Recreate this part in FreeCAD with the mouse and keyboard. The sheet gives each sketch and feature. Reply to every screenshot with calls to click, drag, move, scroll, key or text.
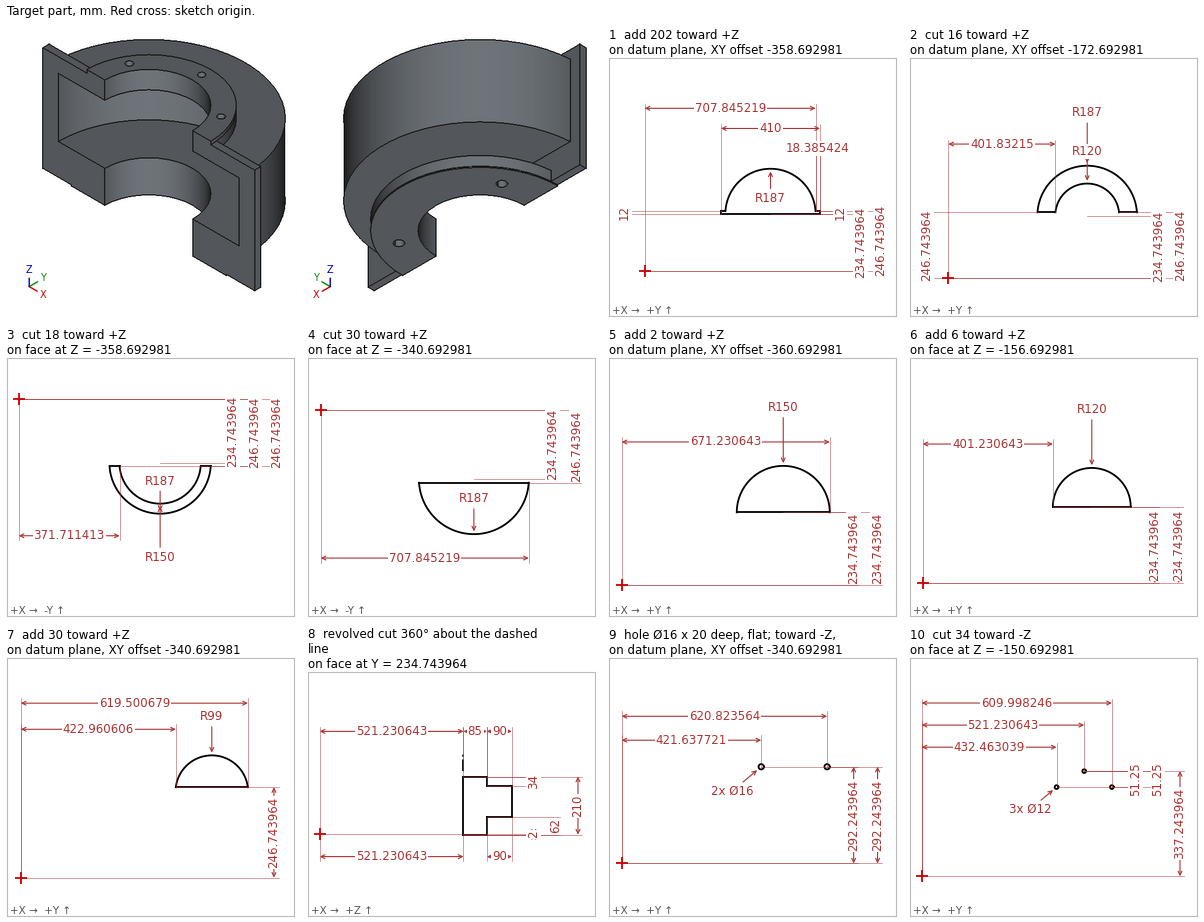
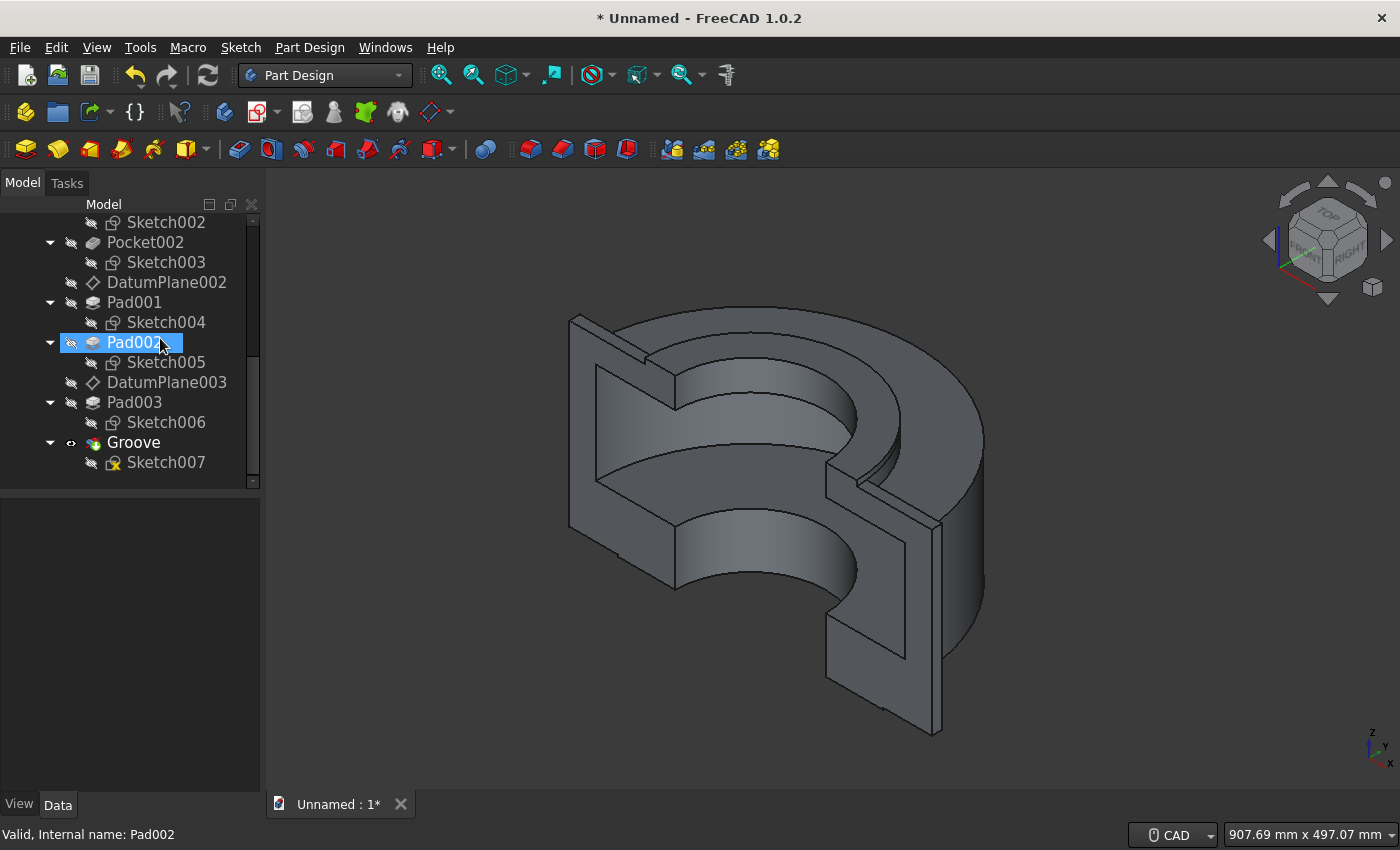
scroll(160, 338, up, 15)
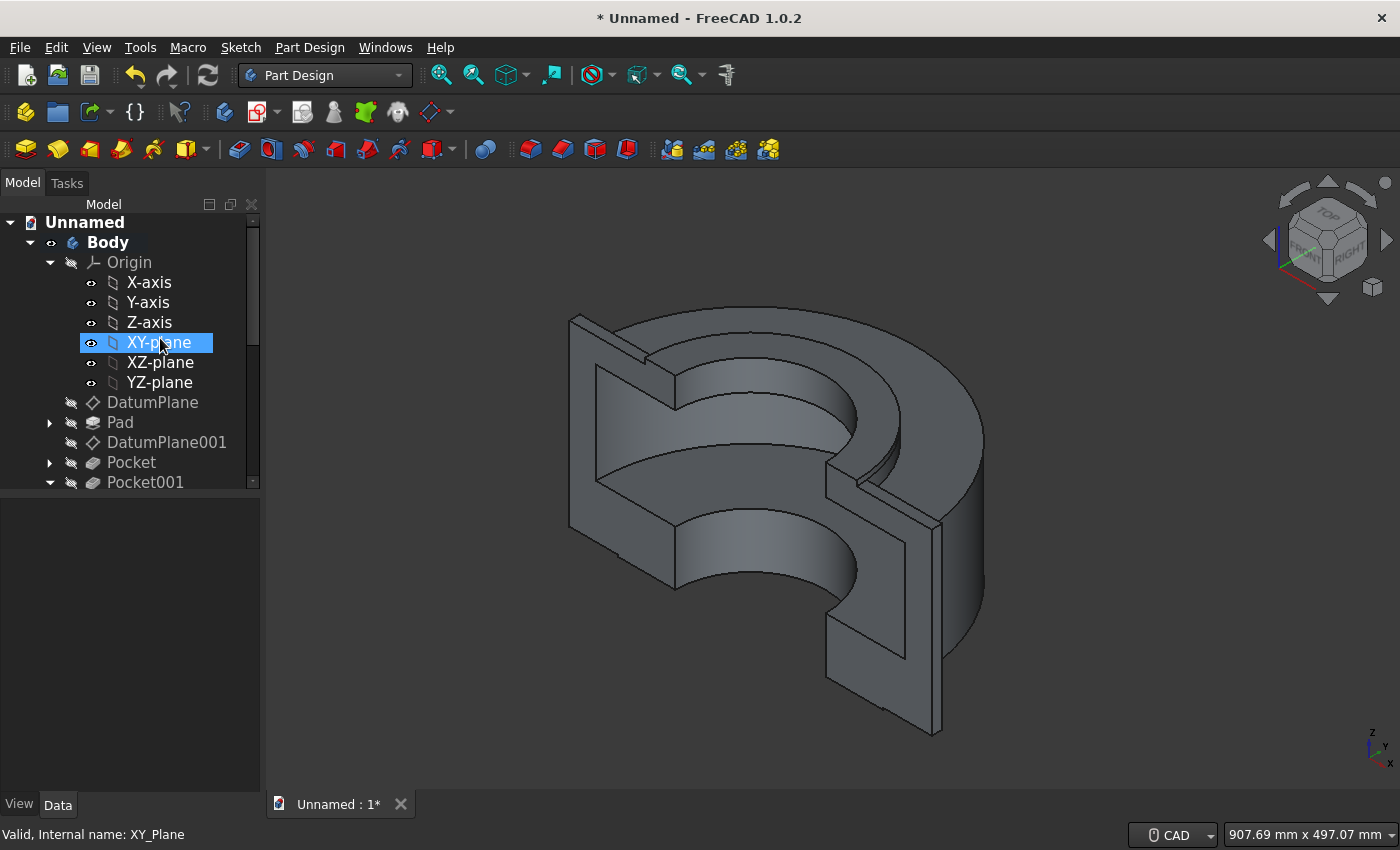
click(136, 343)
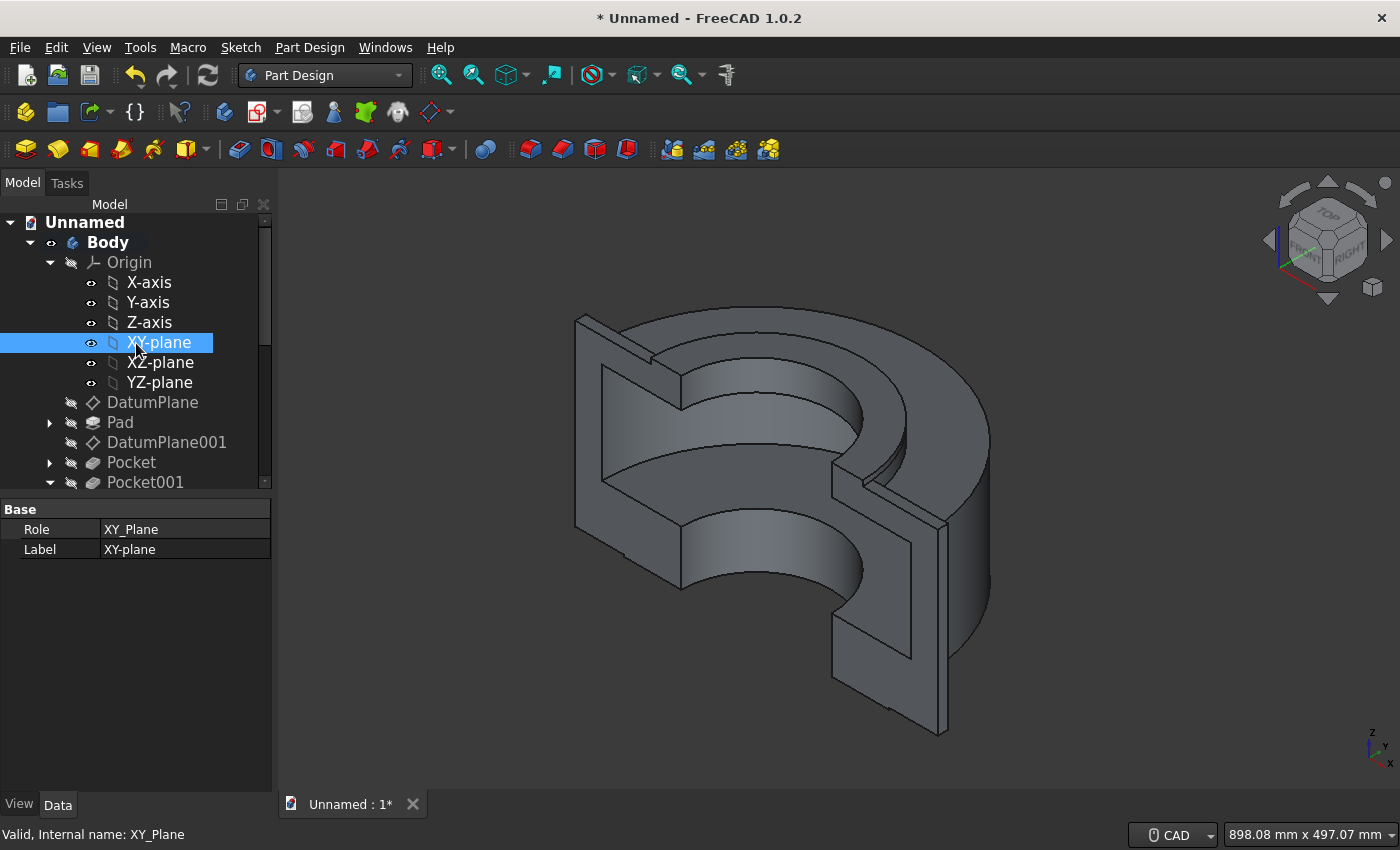
click(430, 112)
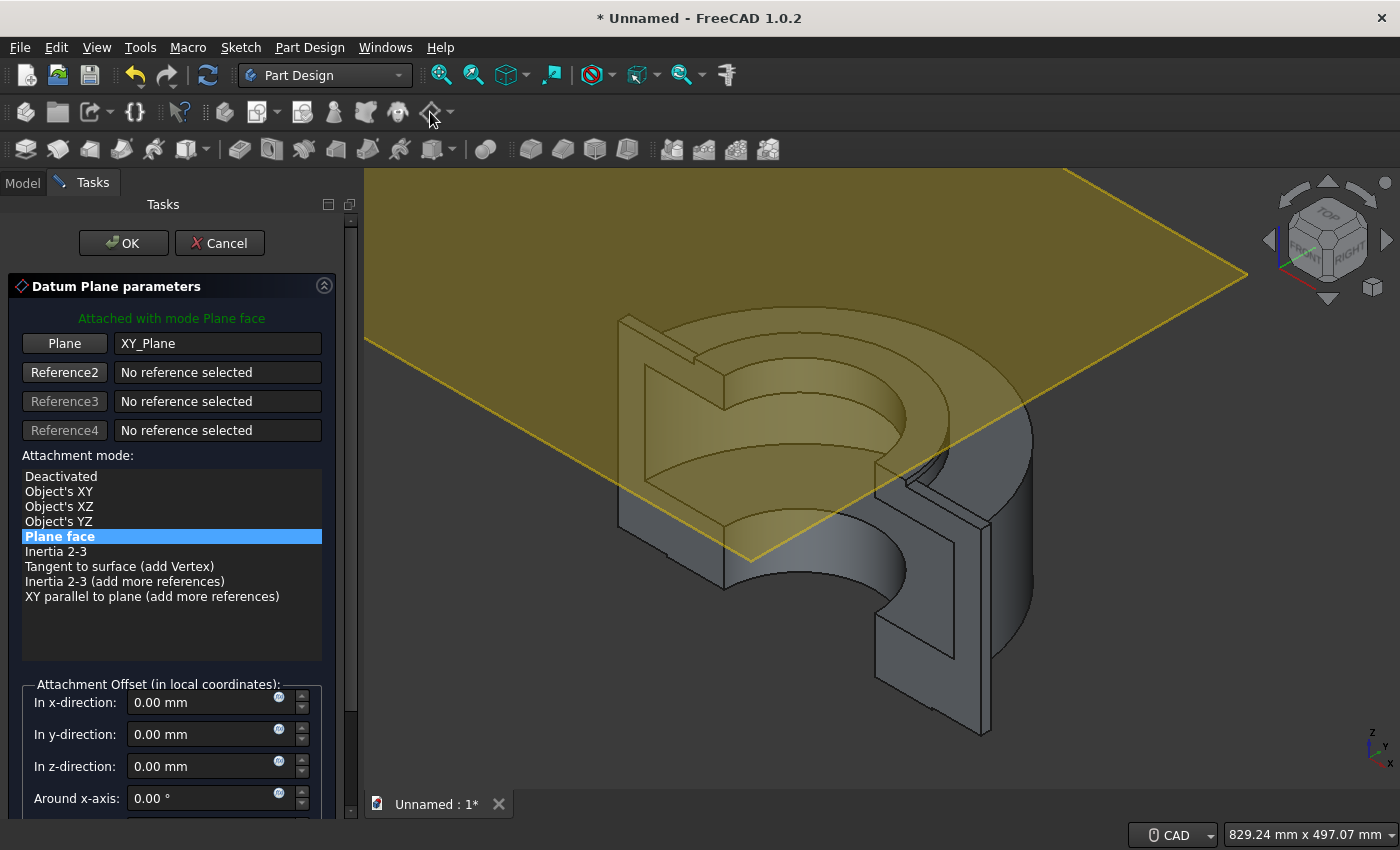
triple_click(210, 766)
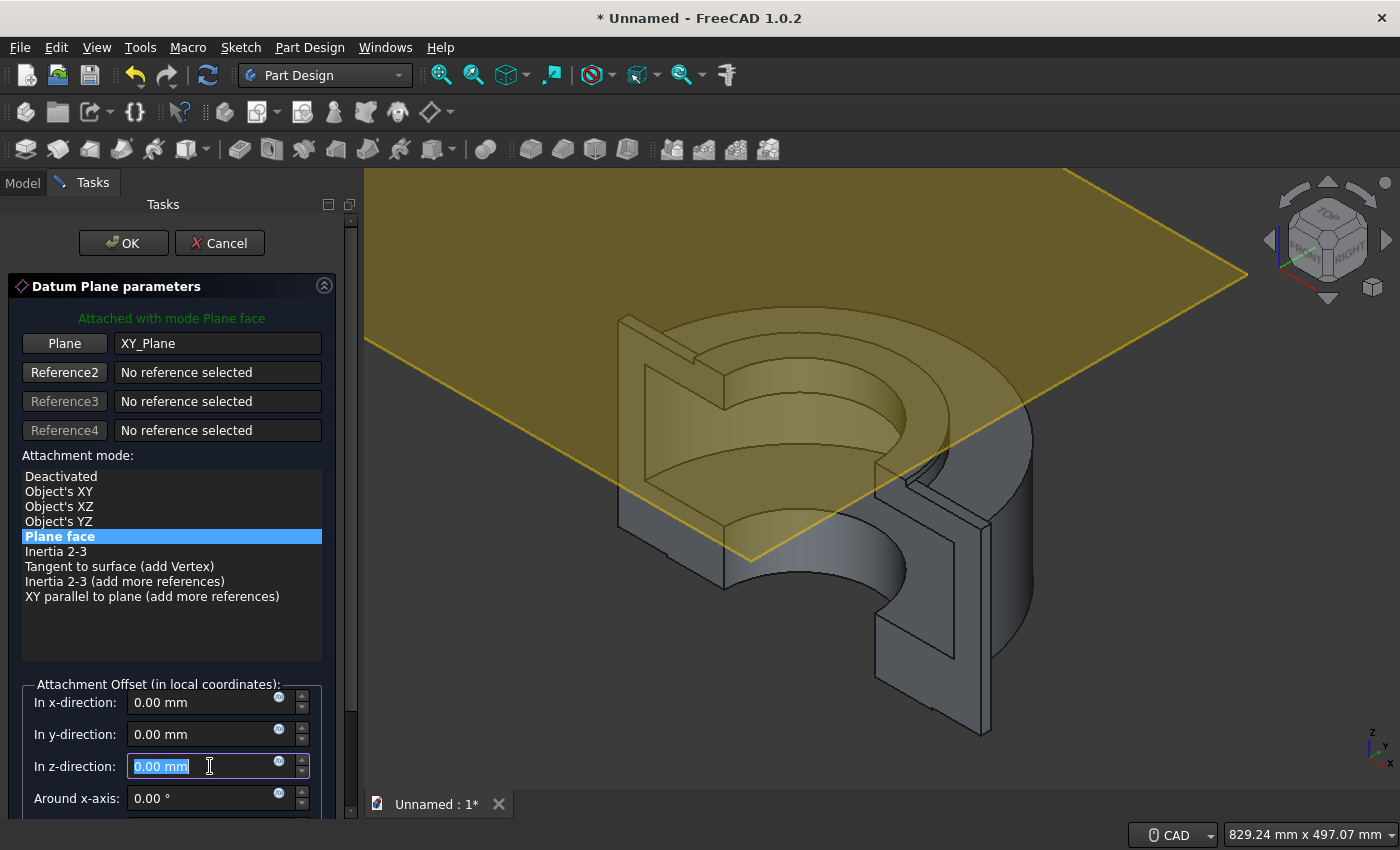
text(-340.692981)
key(Tab)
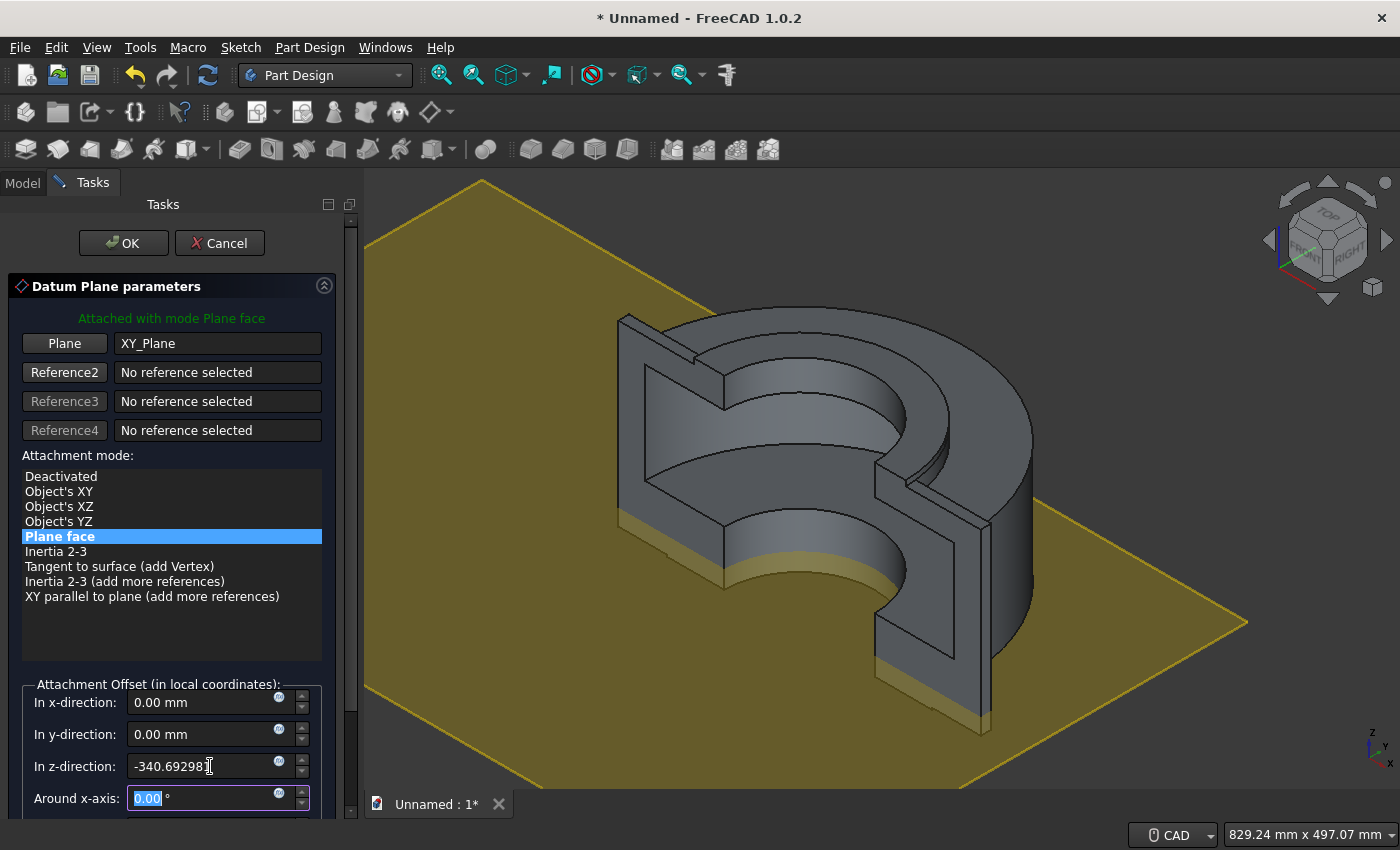
click(124, 243)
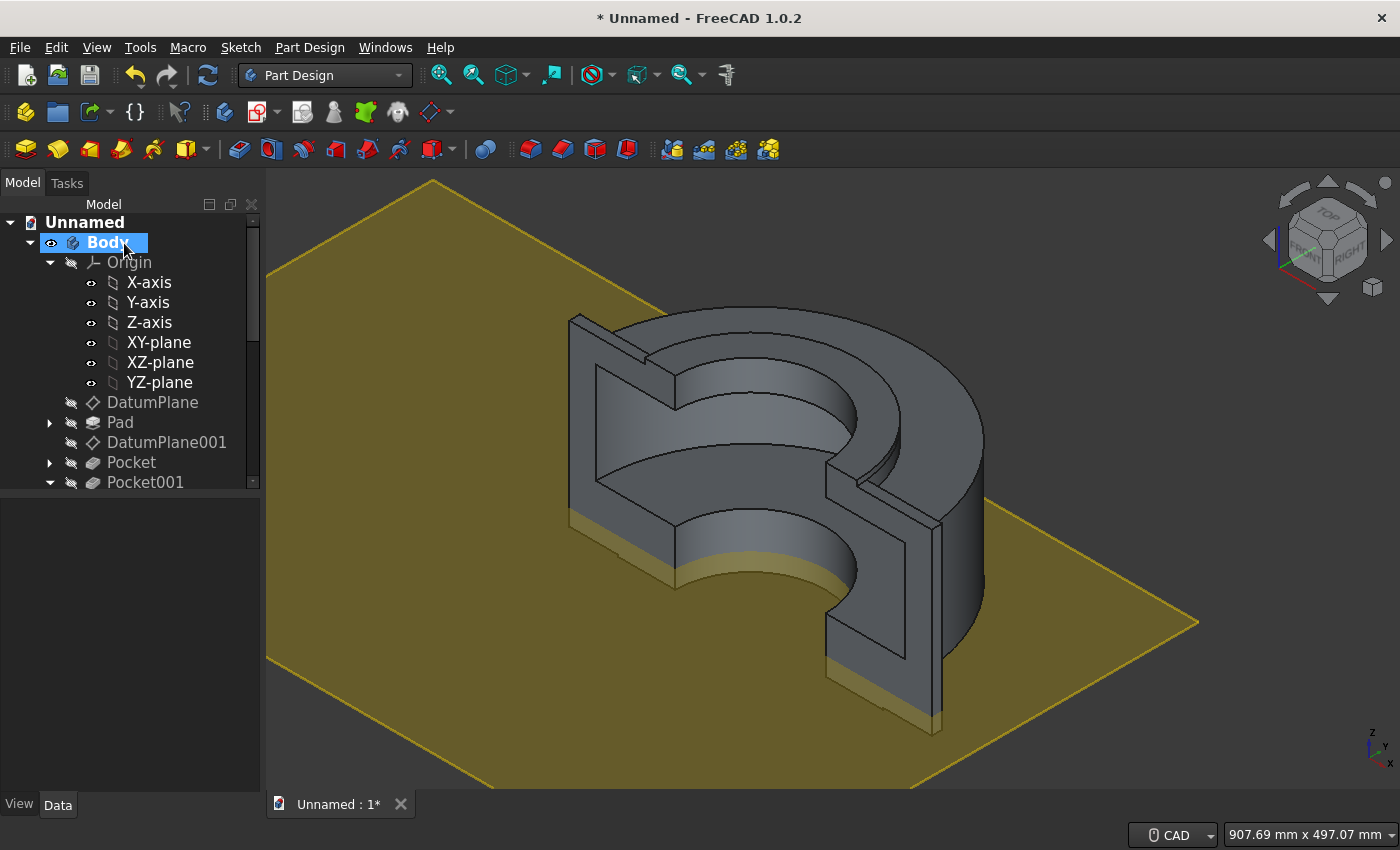
scroll(100, 358, down, 3)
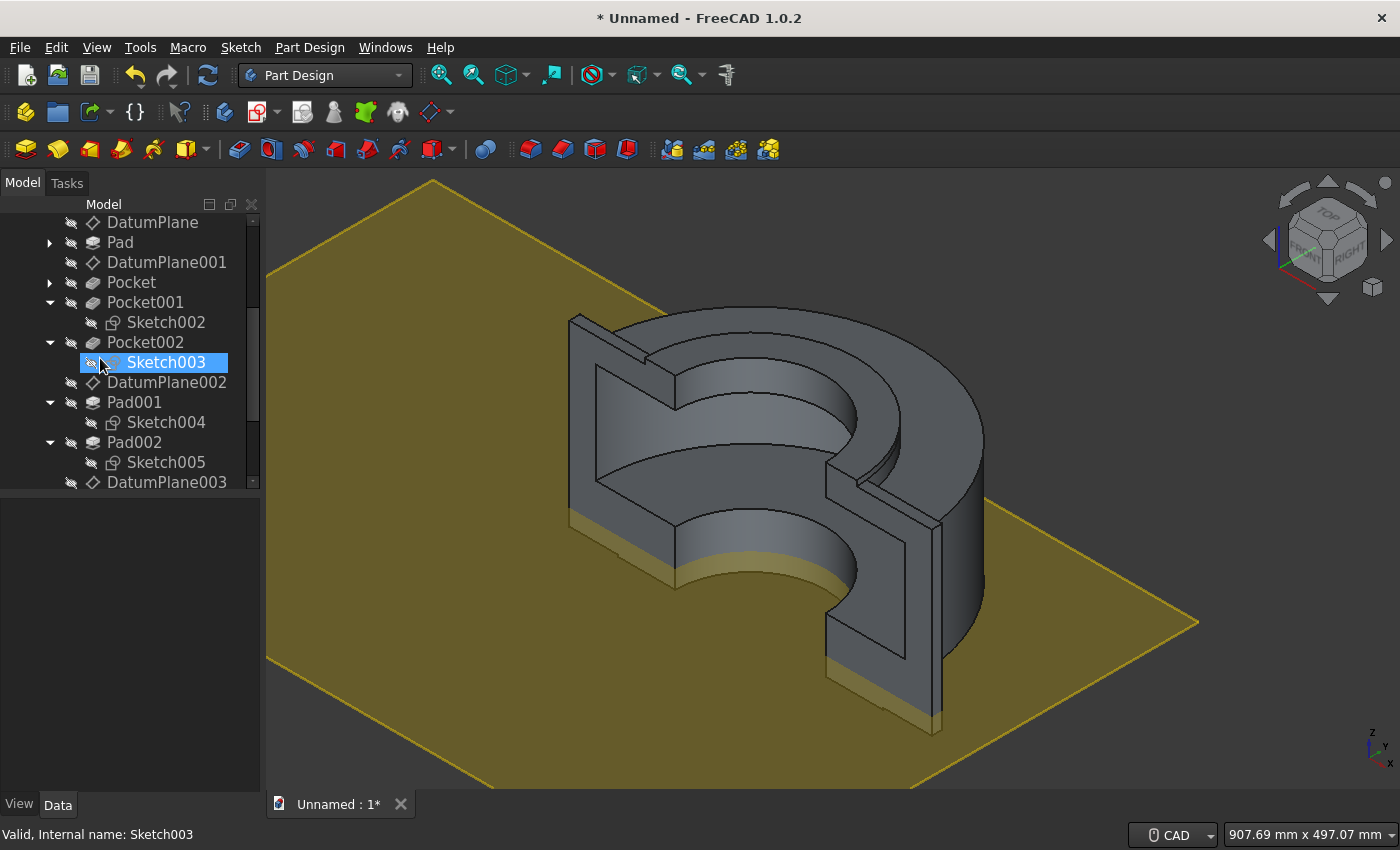
scroll(140, 358, up, 15)